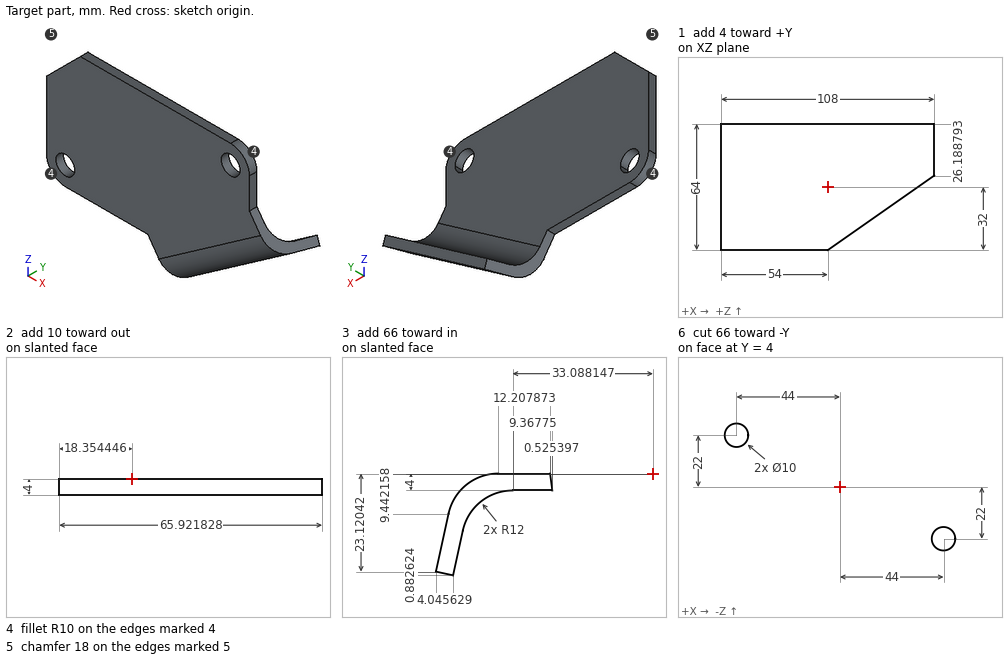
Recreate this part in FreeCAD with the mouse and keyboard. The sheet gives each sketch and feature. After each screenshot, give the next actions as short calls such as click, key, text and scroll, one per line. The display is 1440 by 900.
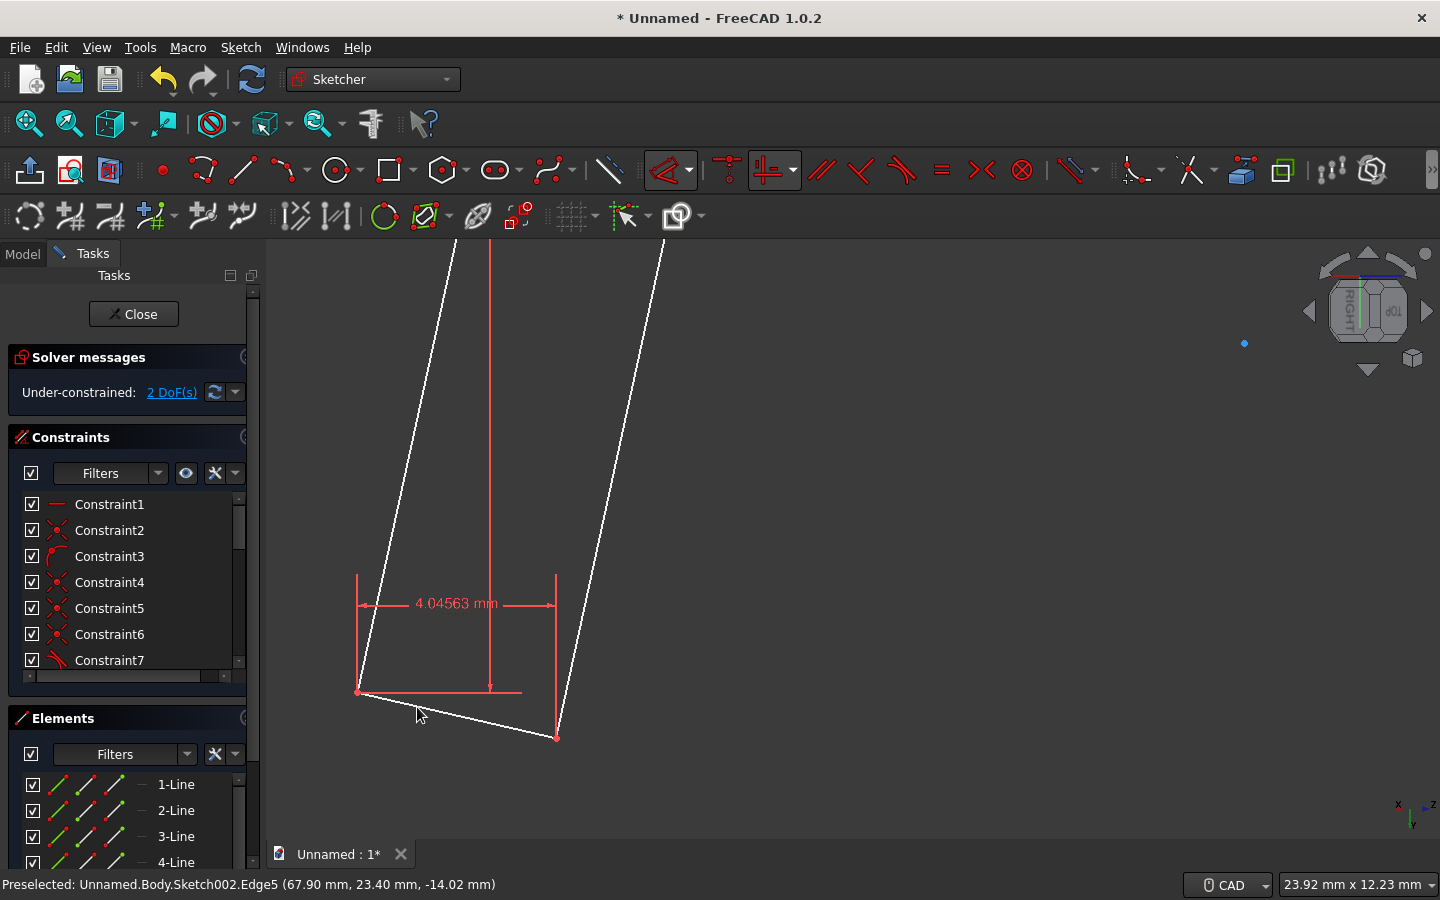
click(417, 706)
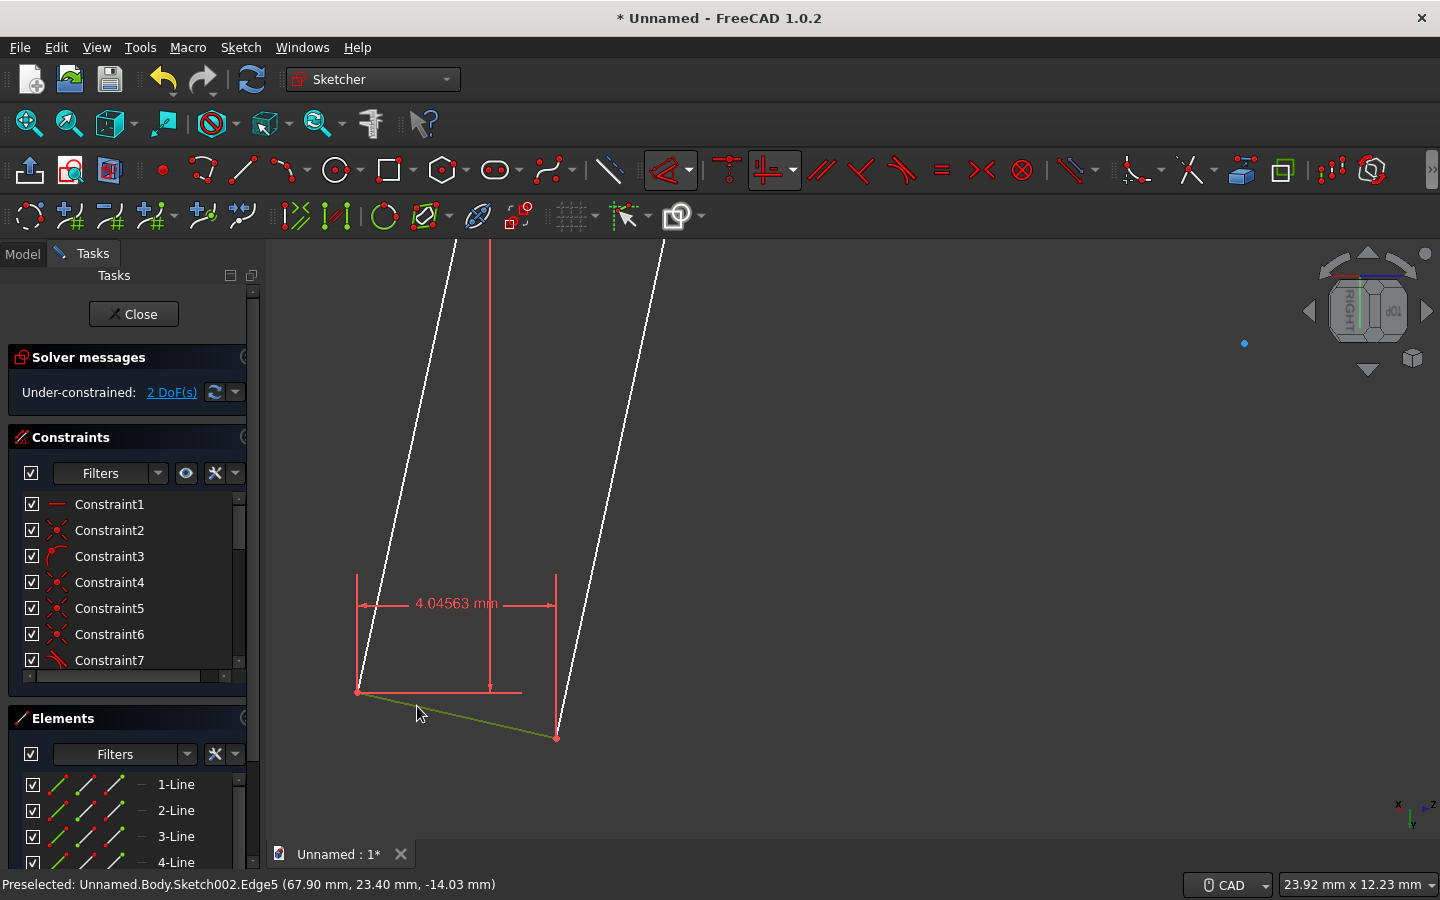
click(692, 170)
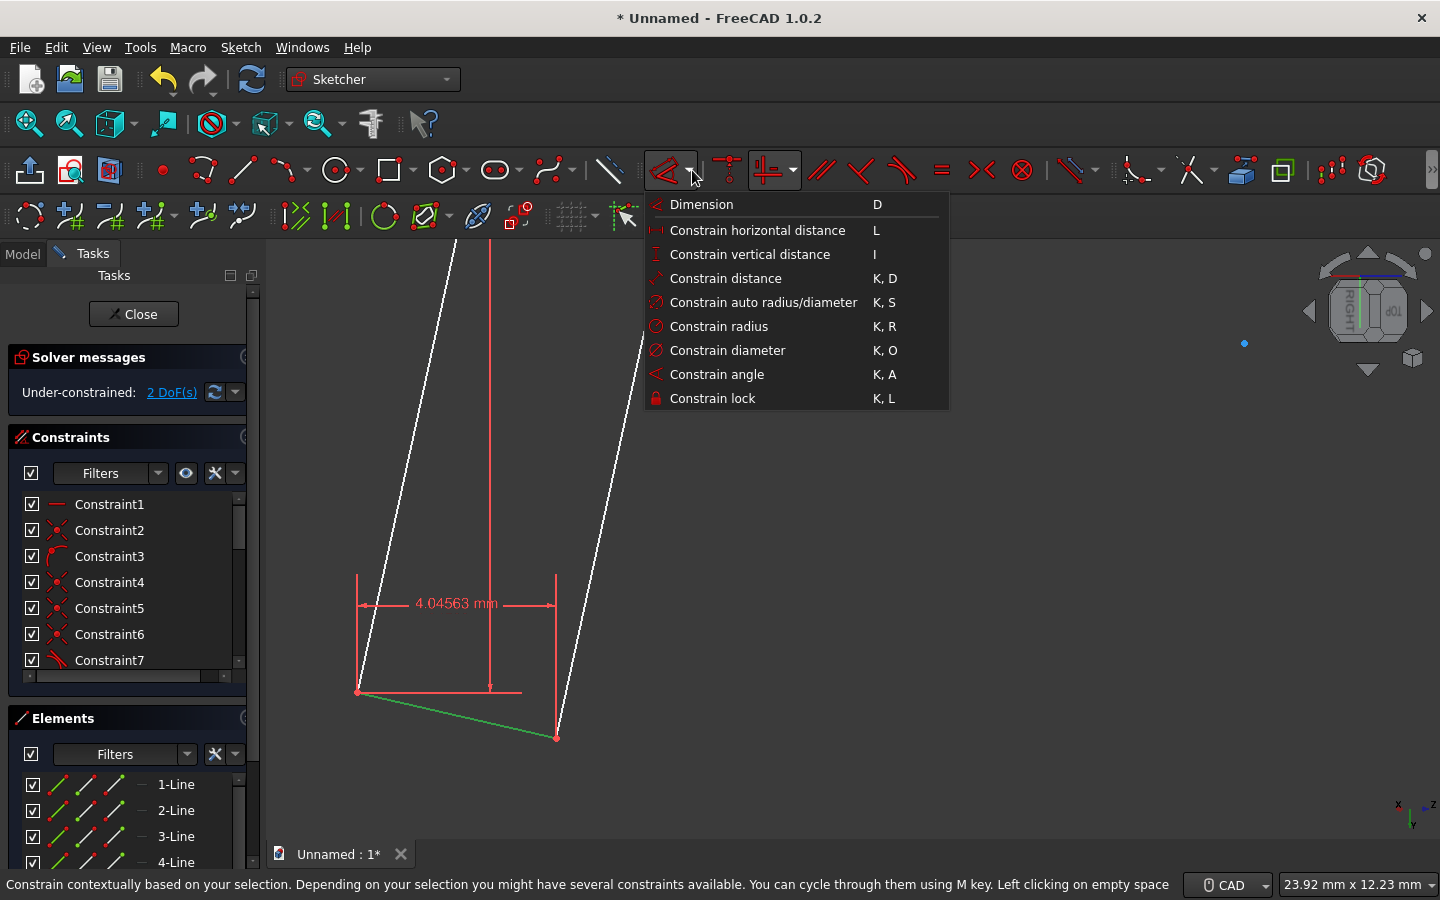
click(797, 254)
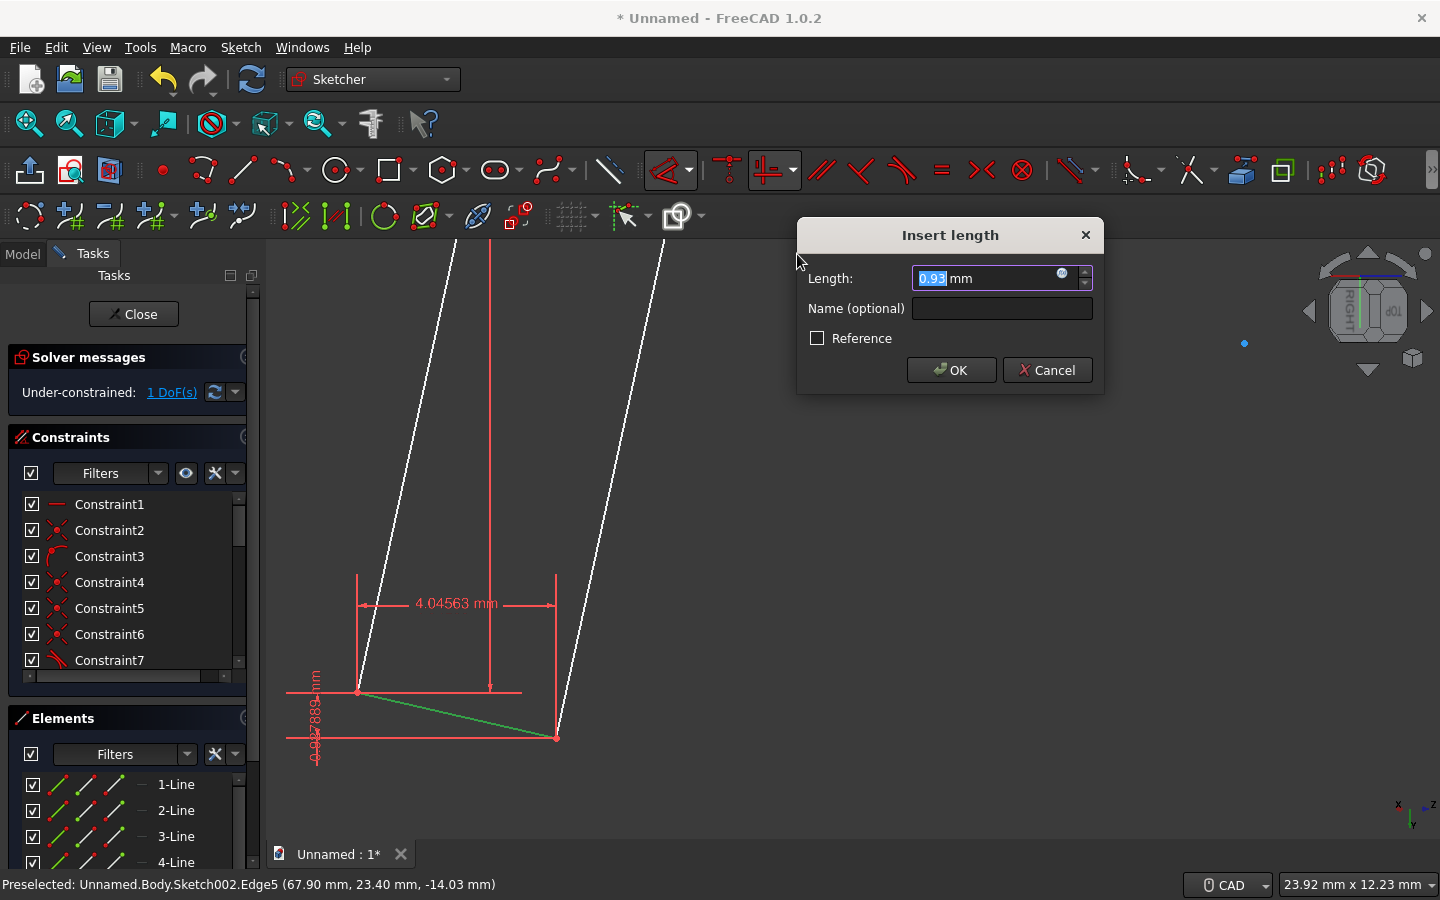
text(0.882624)
key(Return)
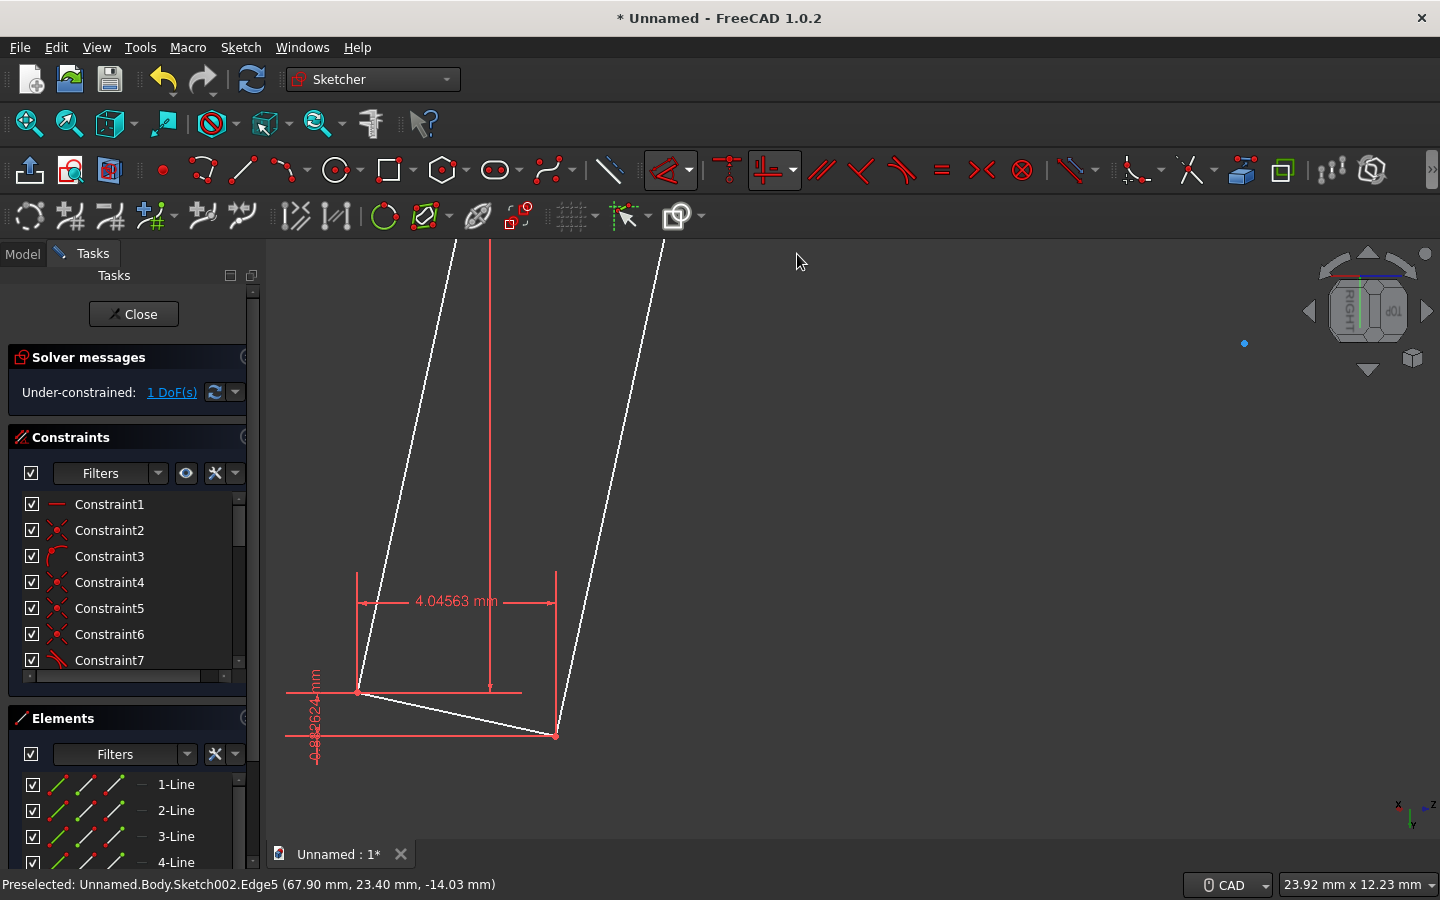
scroll(417, 708, down, 6)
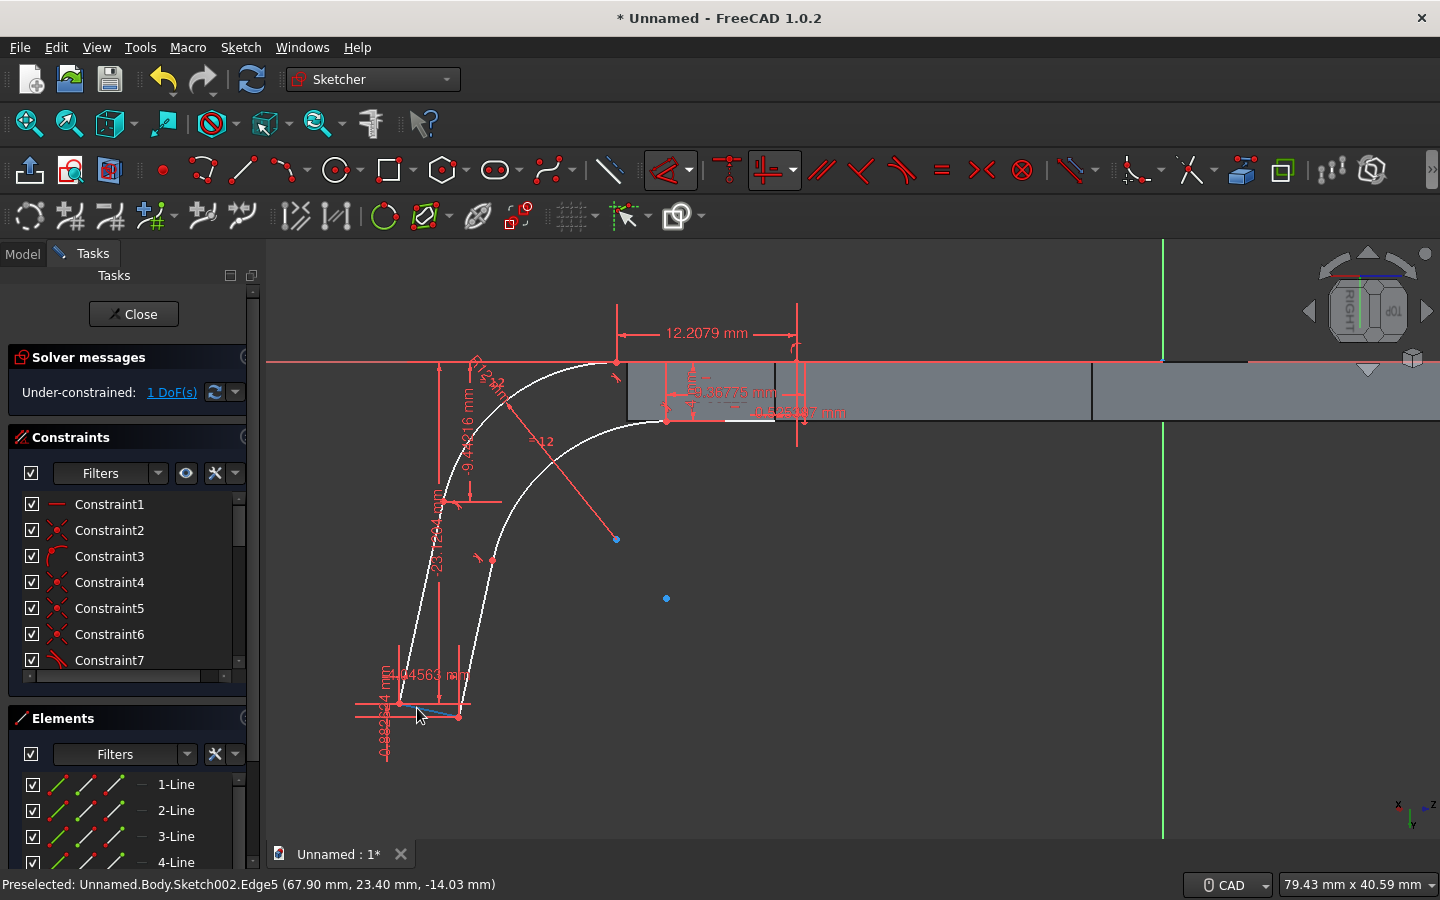
click(666, 421)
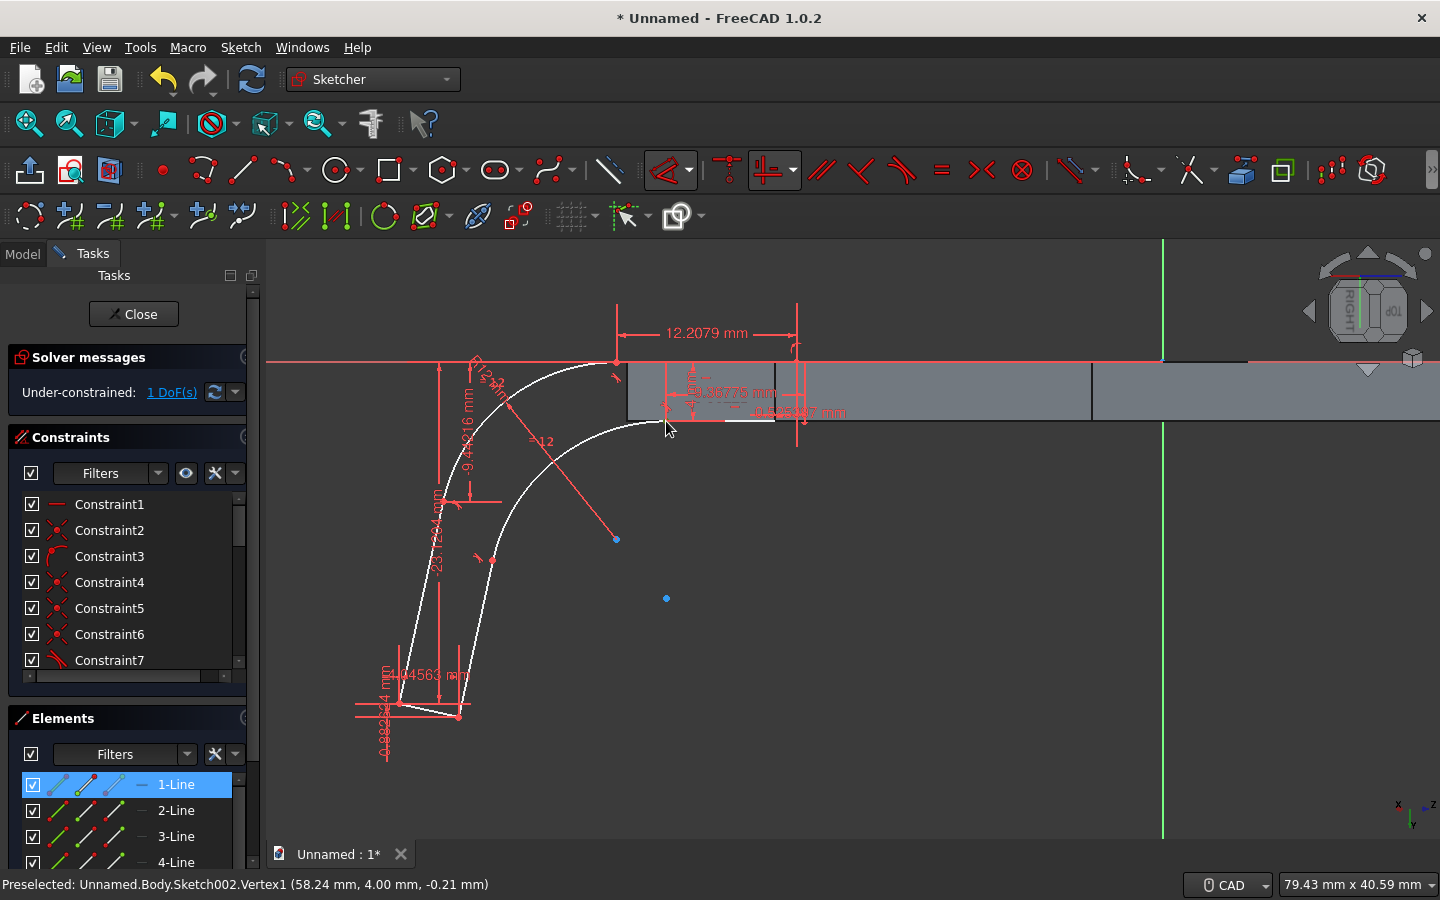
key(l)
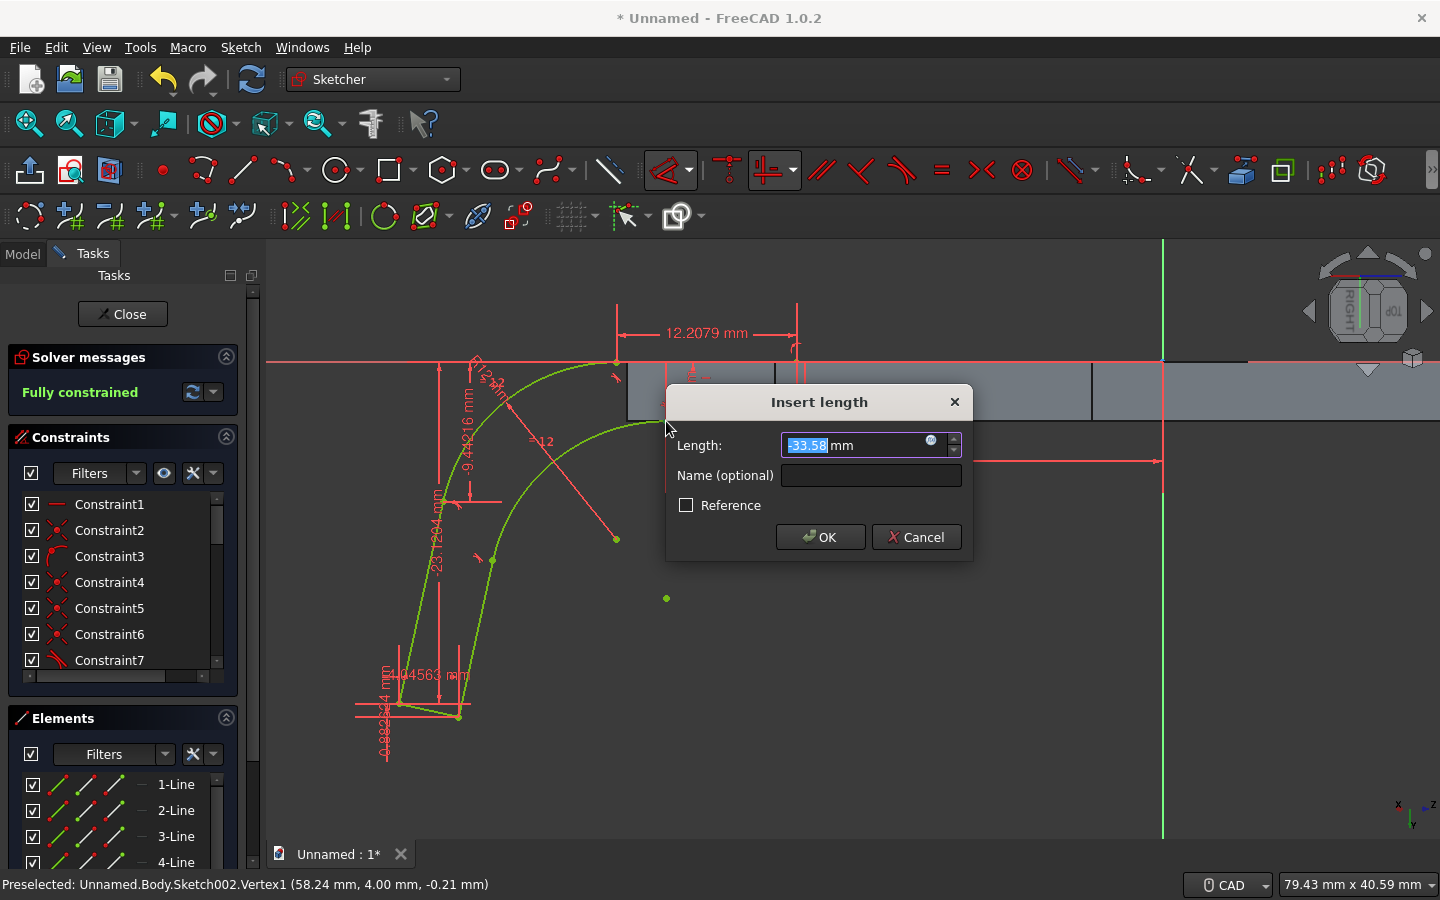
text(-33.088147)
key(Return)